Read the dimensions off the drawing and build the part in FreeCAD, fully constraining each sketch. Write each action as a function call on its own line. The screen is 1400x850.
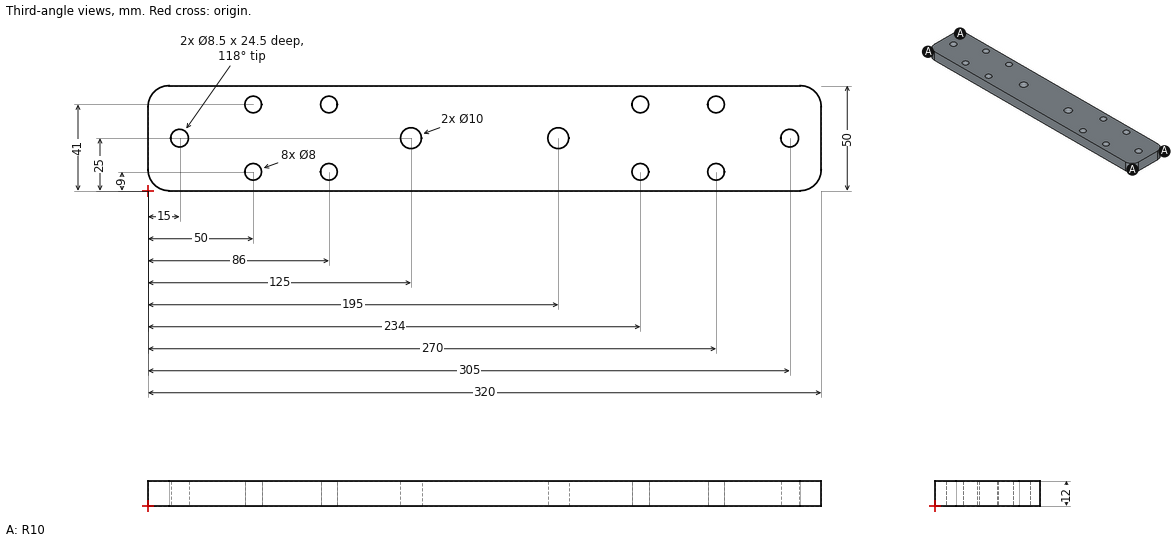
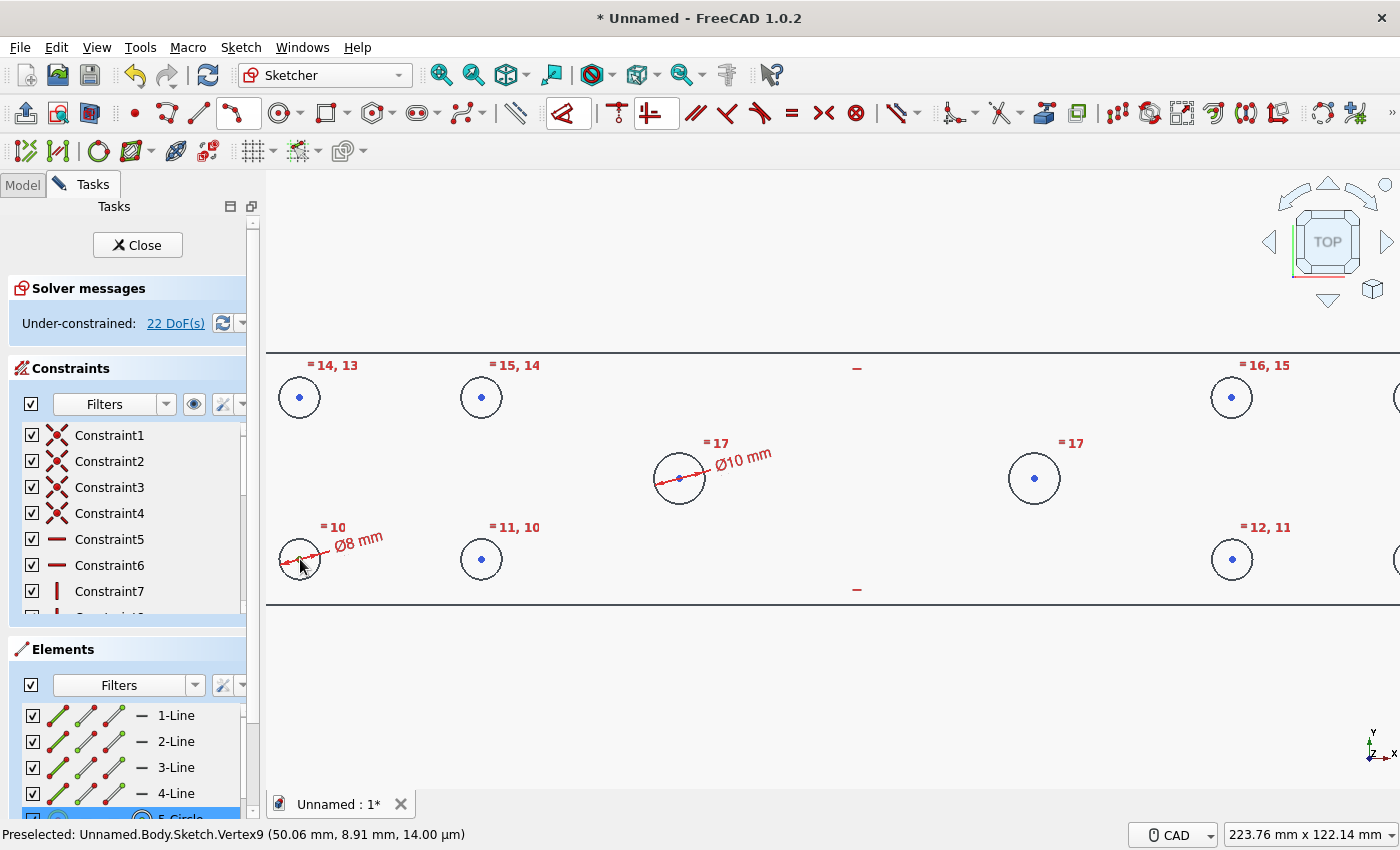
key(i)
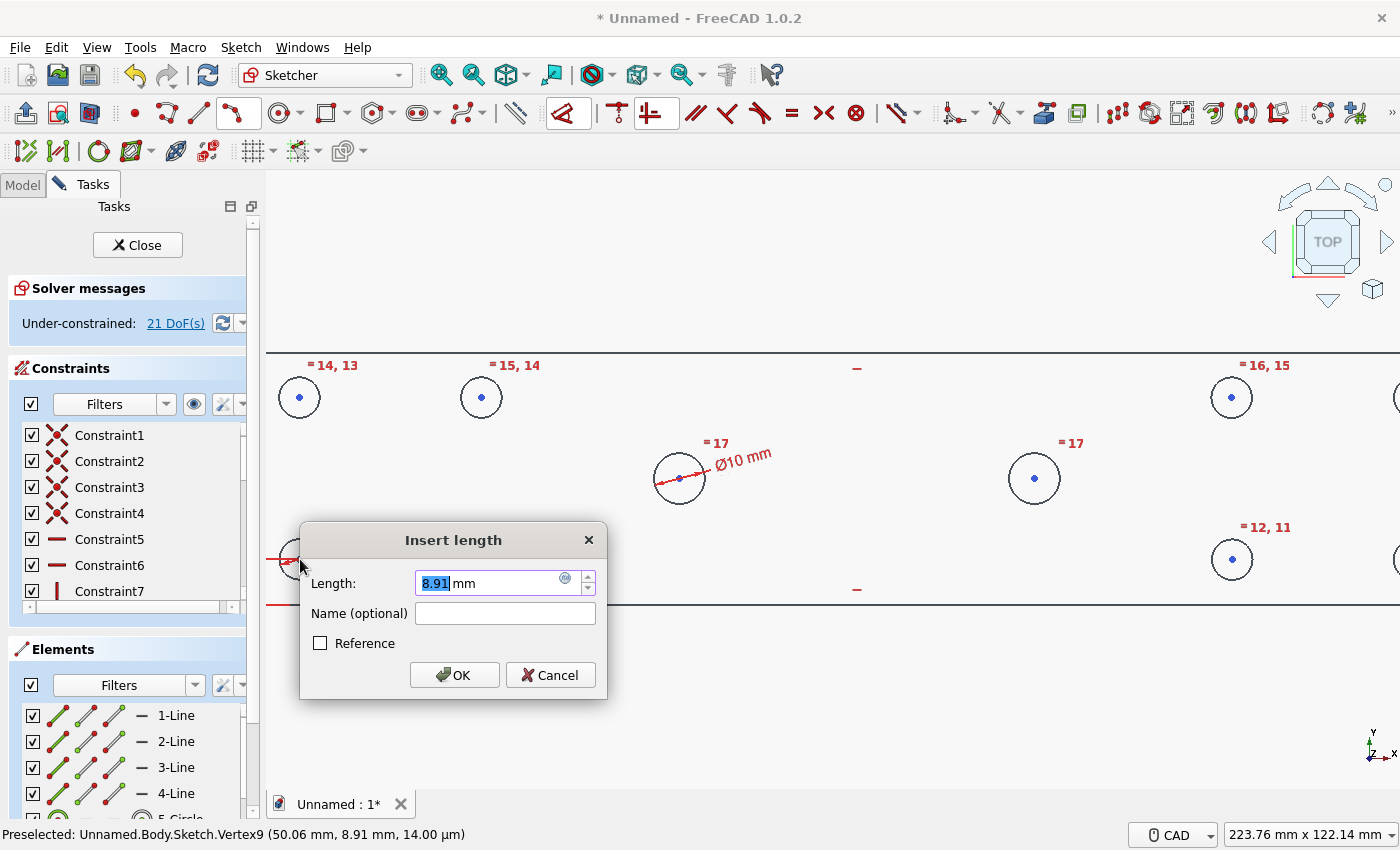
text(9)
key(Return)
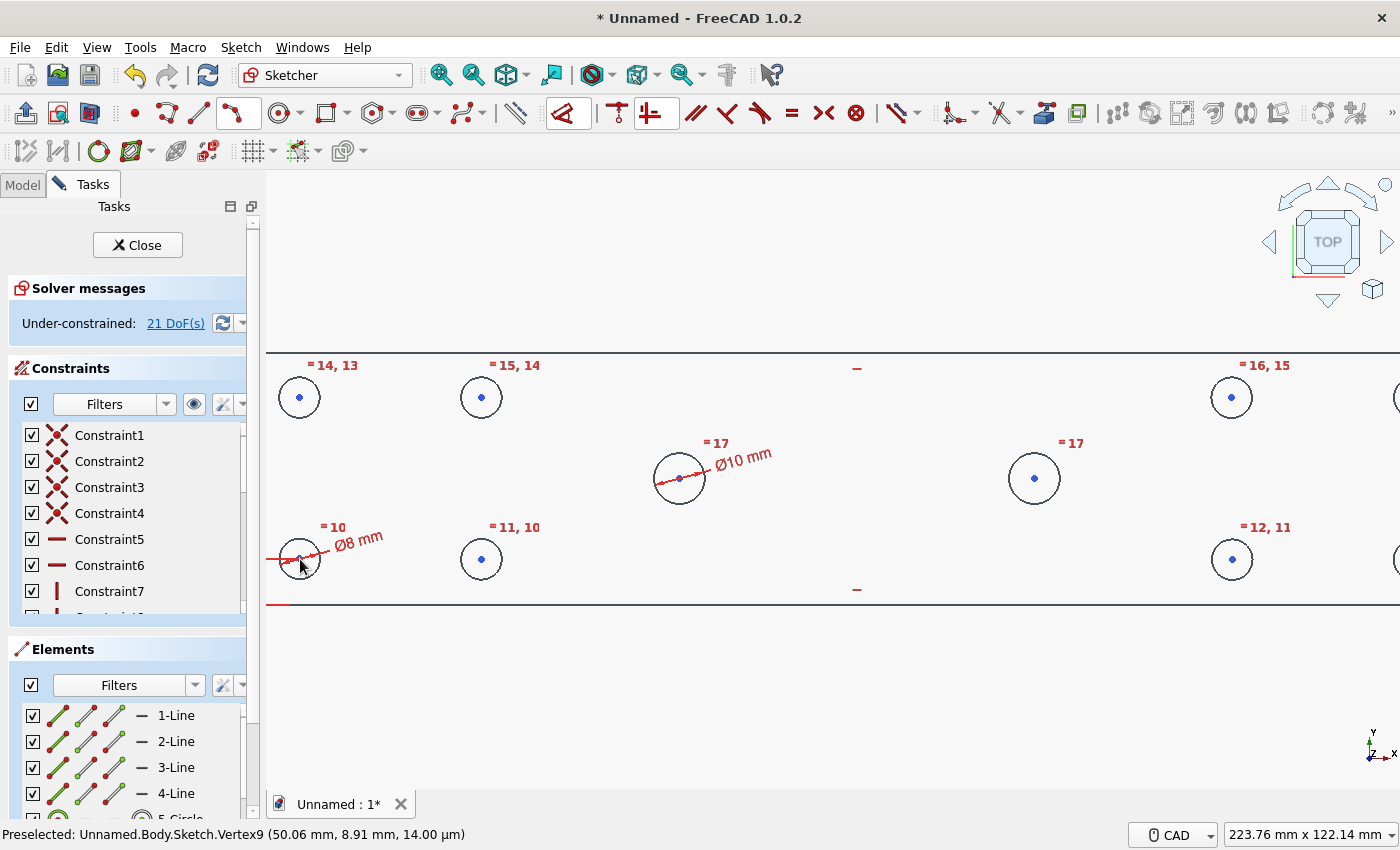
click(481, 559)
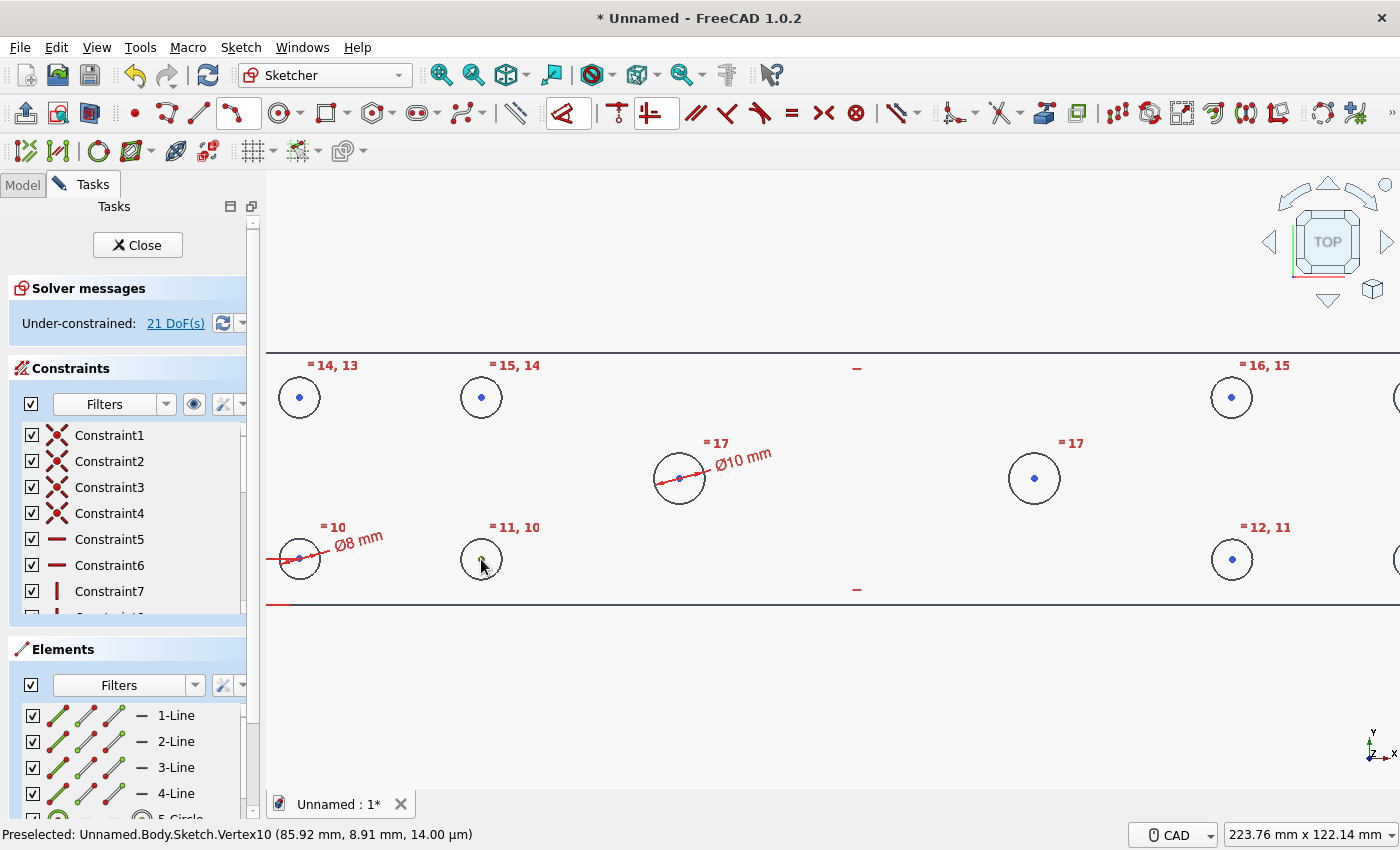
key(i)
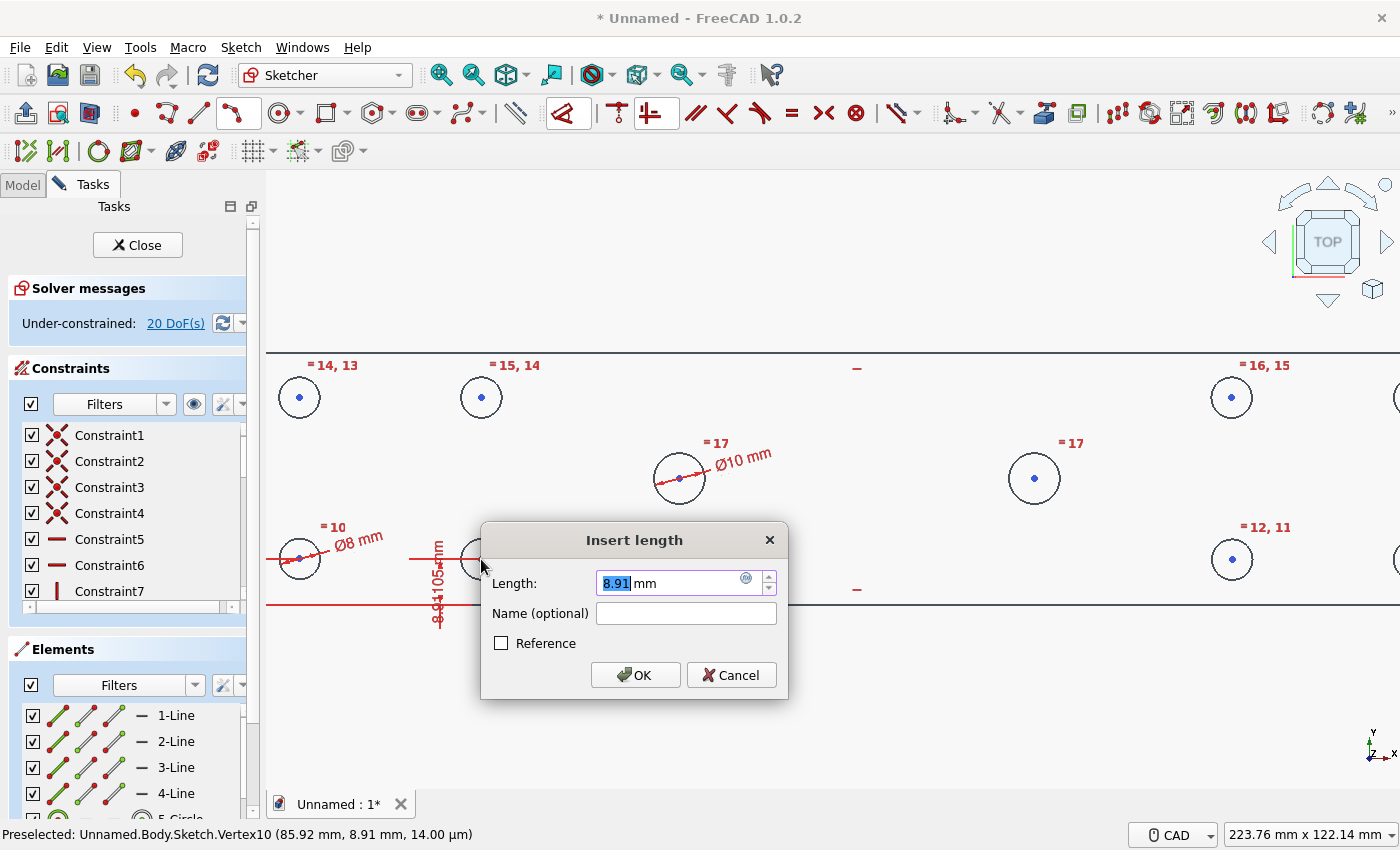
text(9)
key(Return)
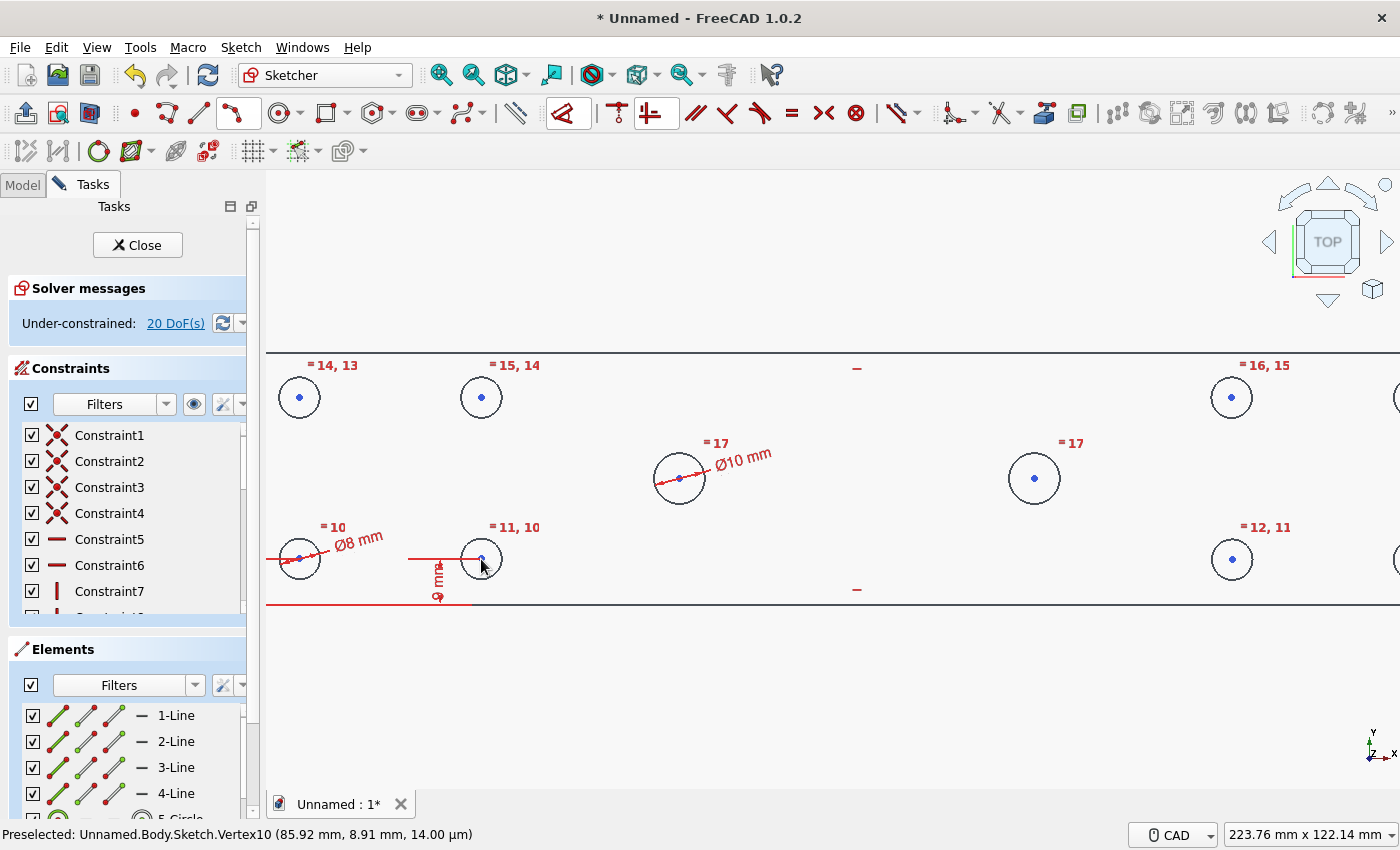
click(1232, 560)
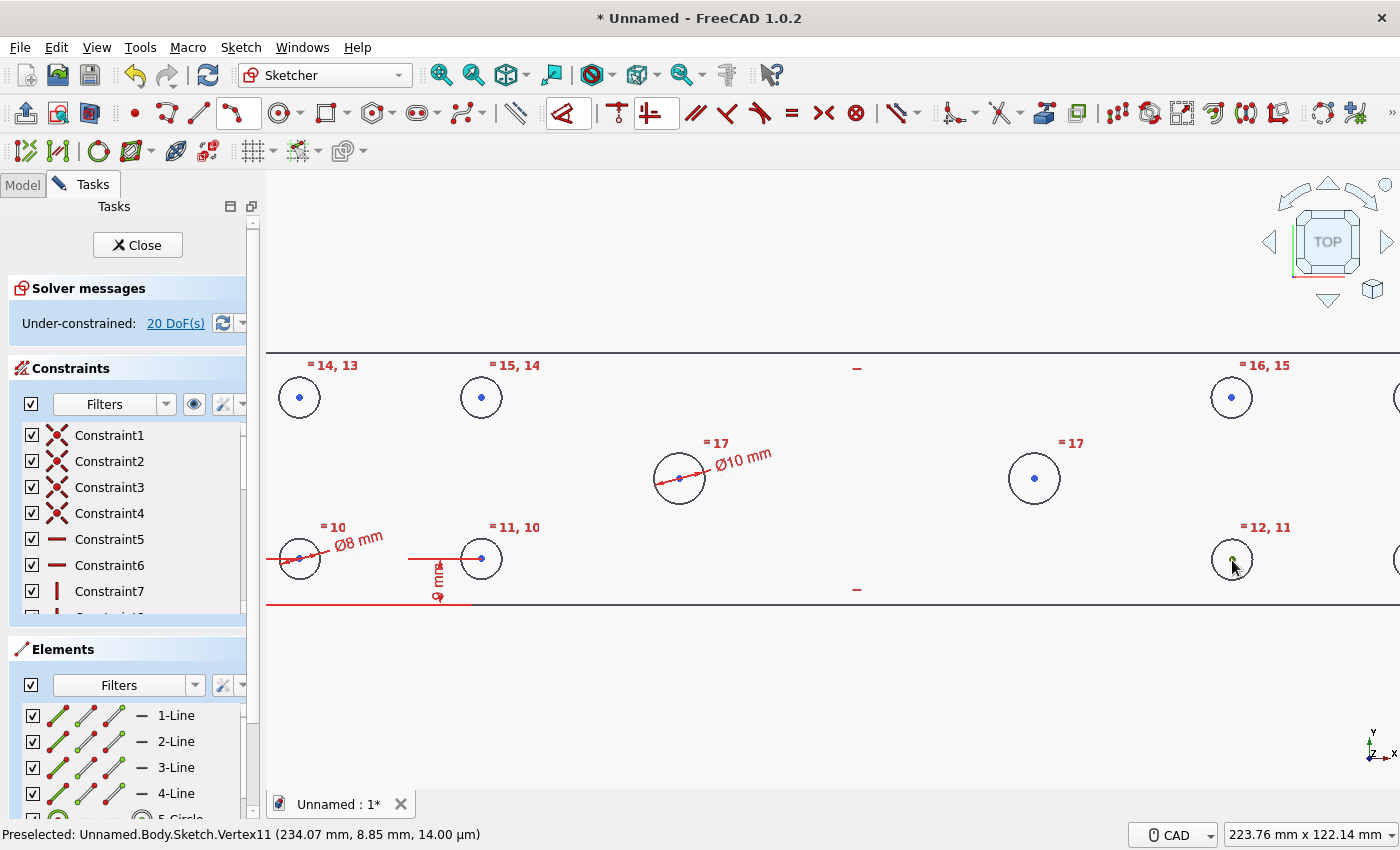
key(i)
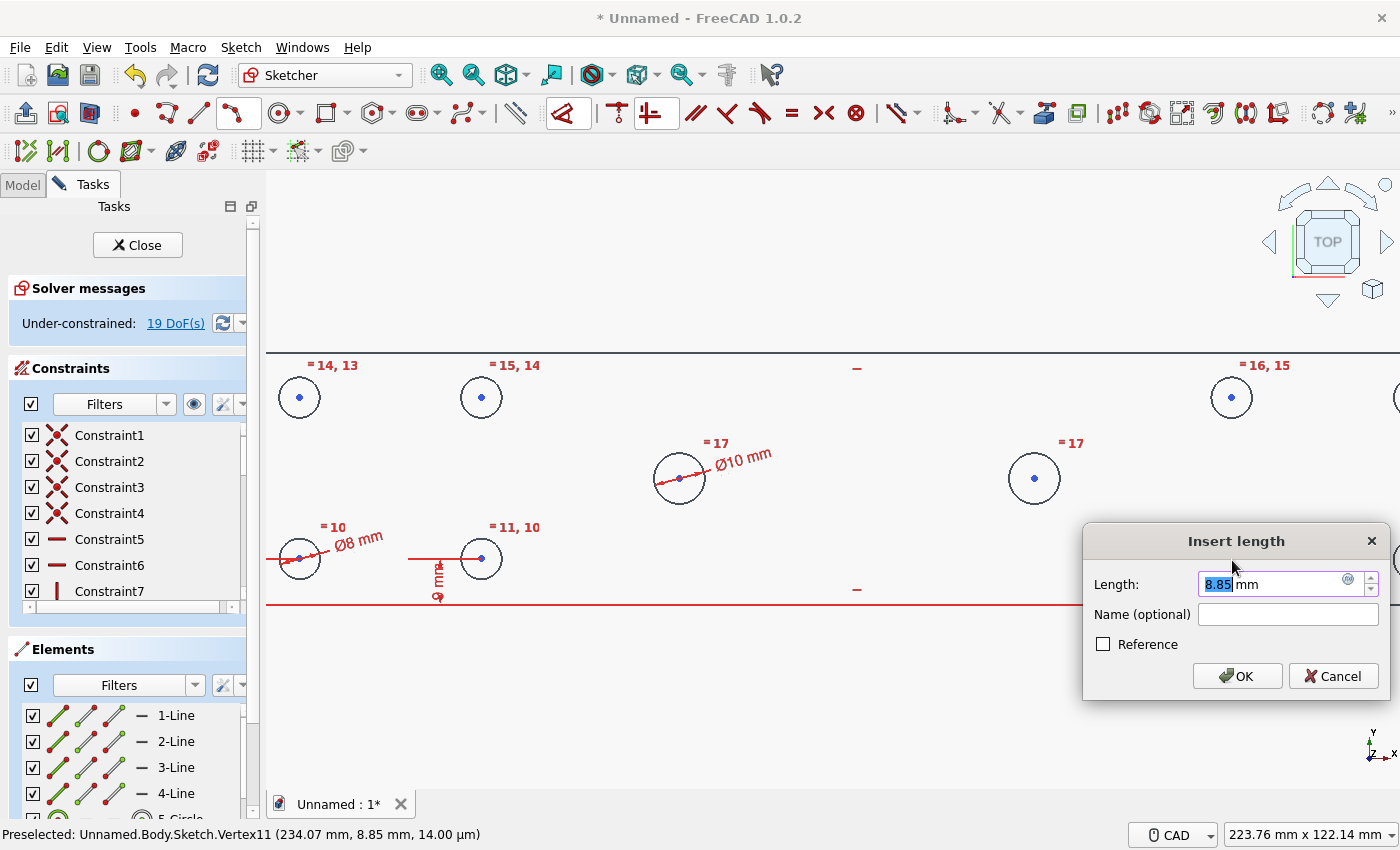
text(9)
key(Return)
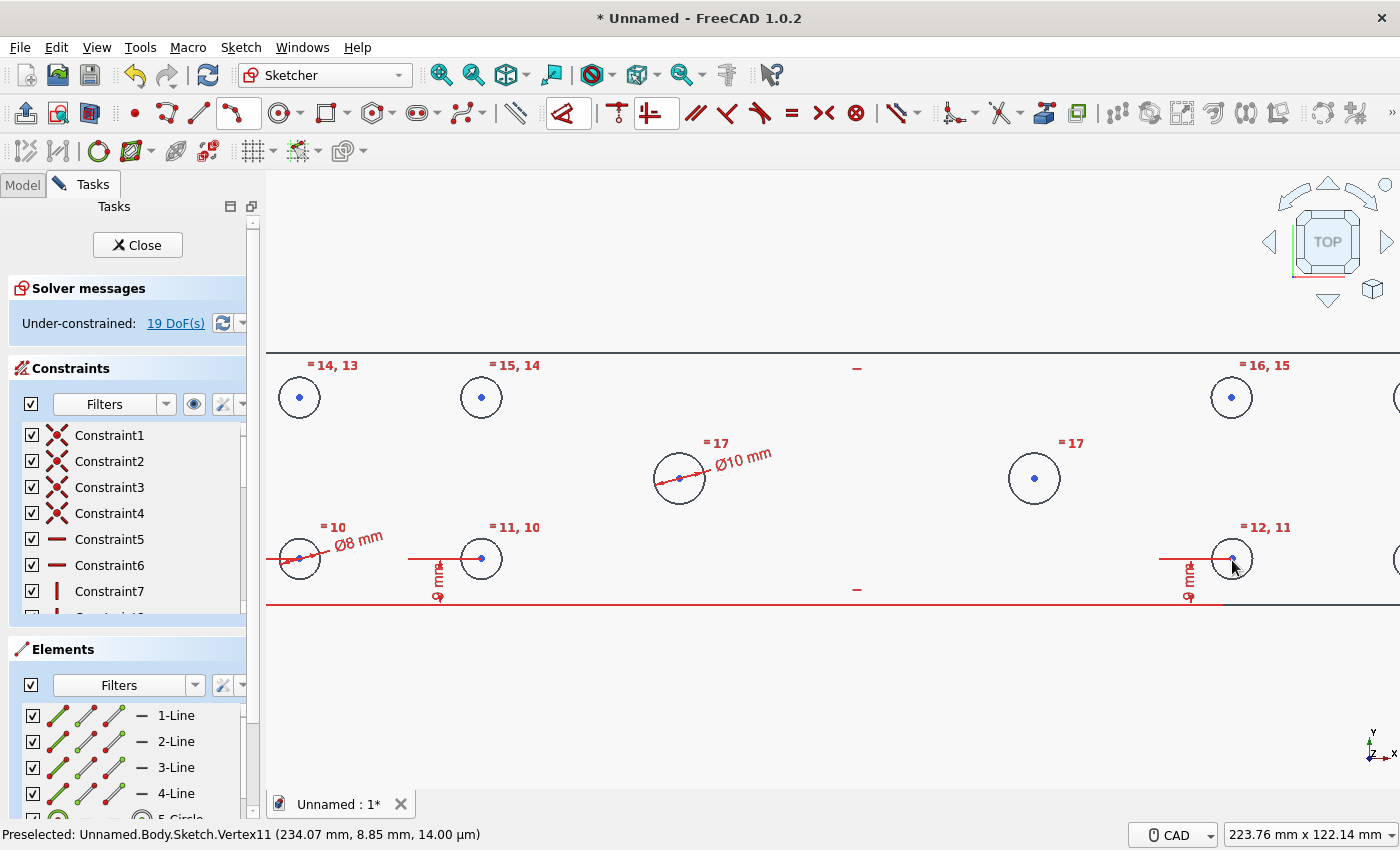
scroll(689, 481, down, 4)